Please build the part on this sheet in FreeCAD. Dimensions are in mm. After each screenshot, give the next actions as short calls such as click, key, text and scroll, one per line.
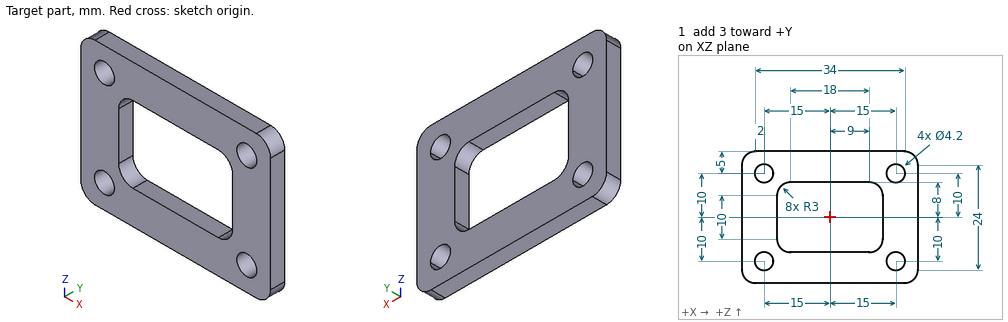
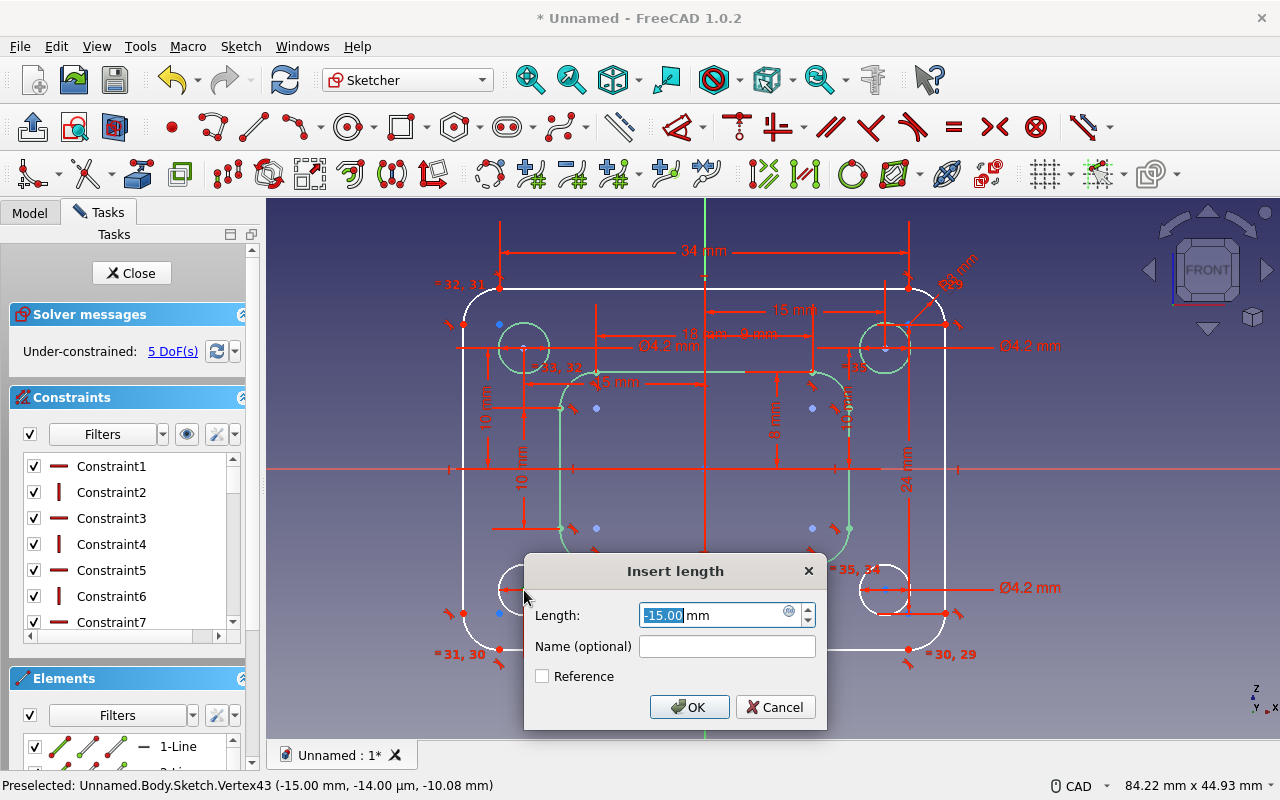
text(-15)
key(Return)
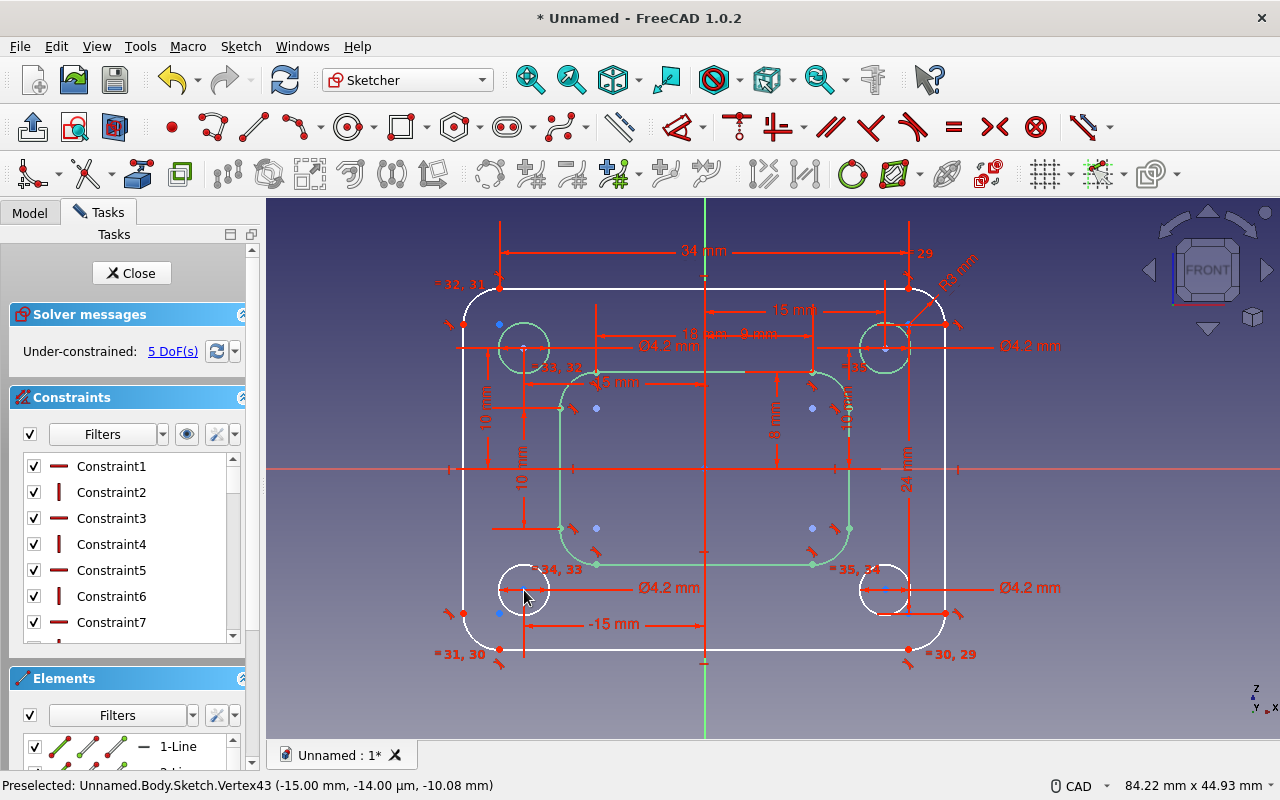
click(524, 590)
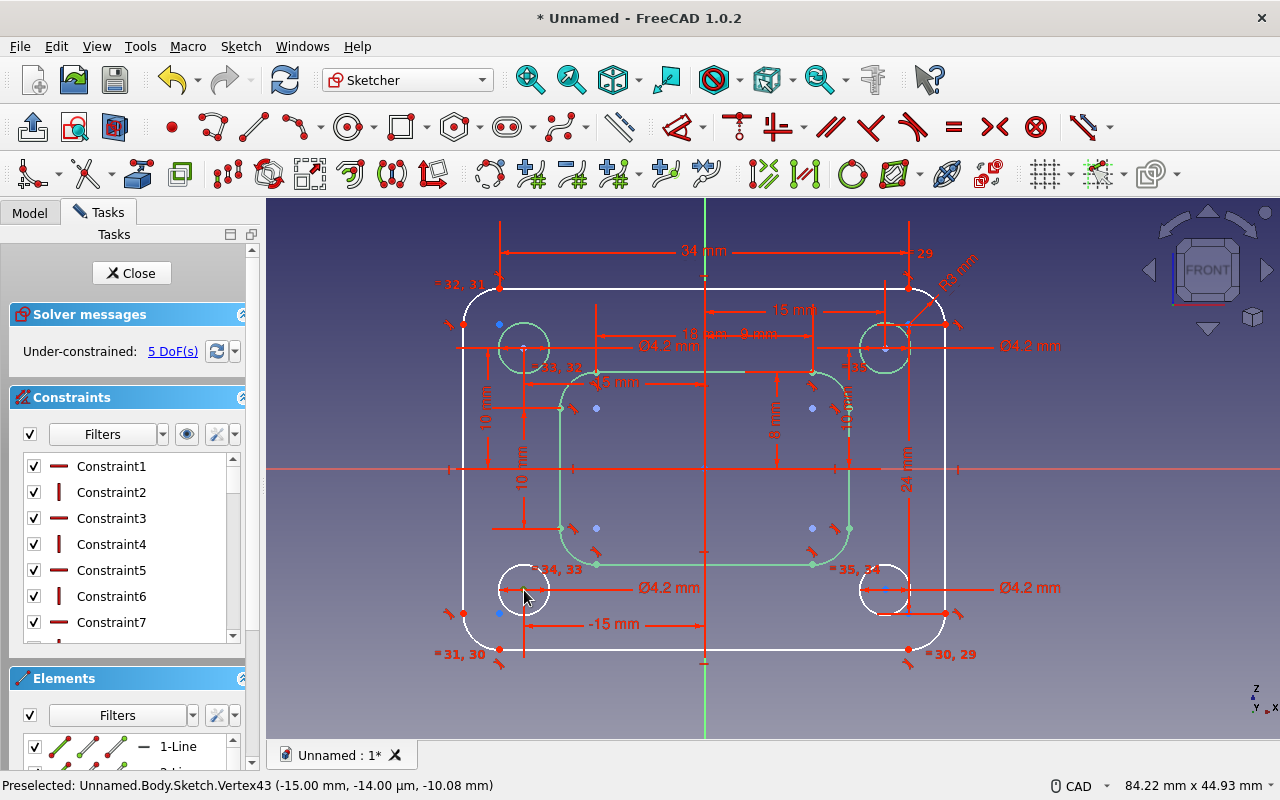
key(i)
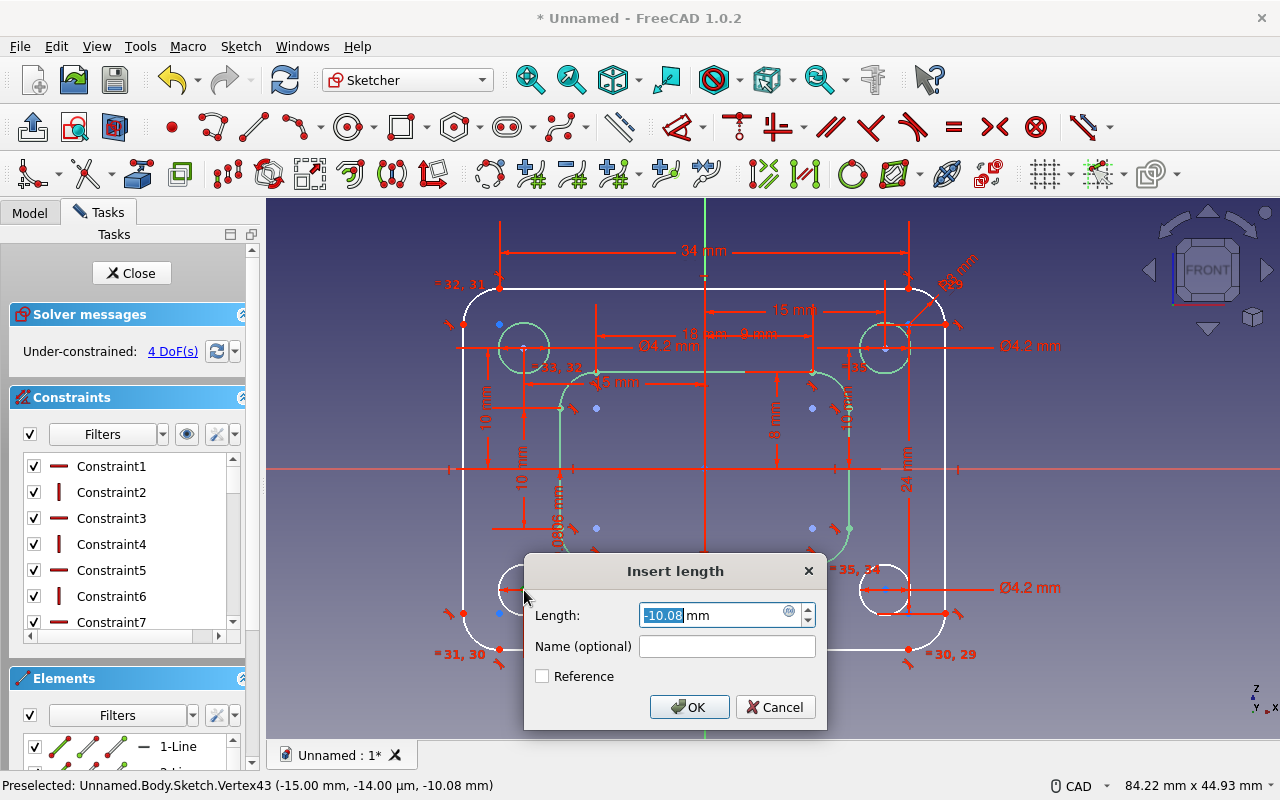
text(-10)
key(Return)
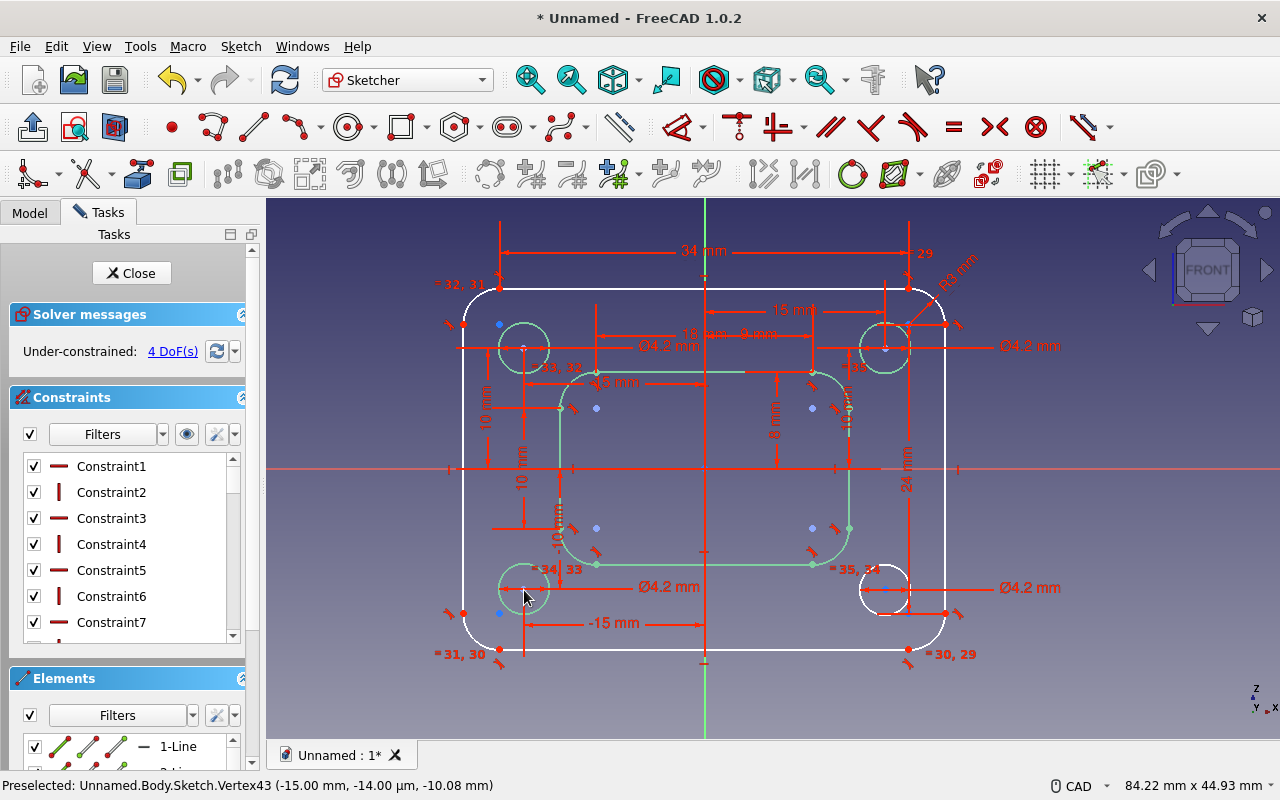
click(885, 590)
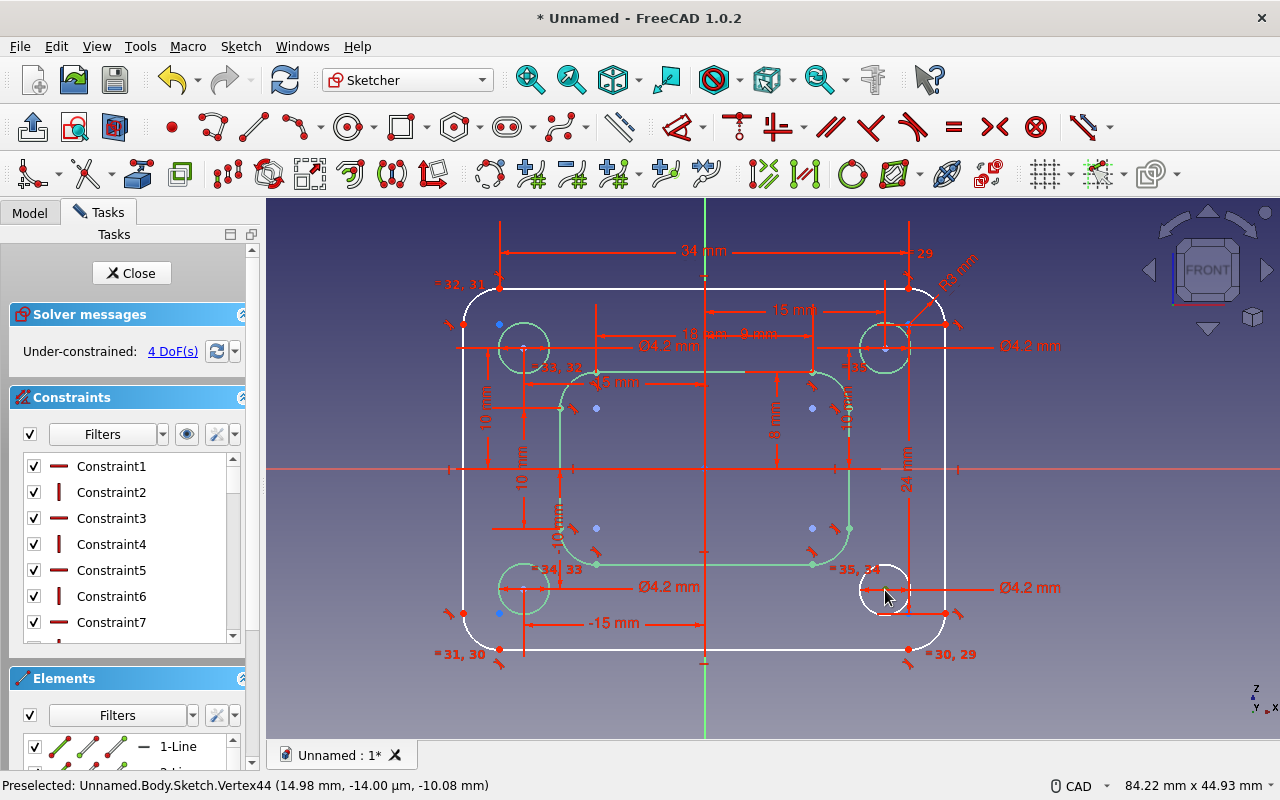
key(l)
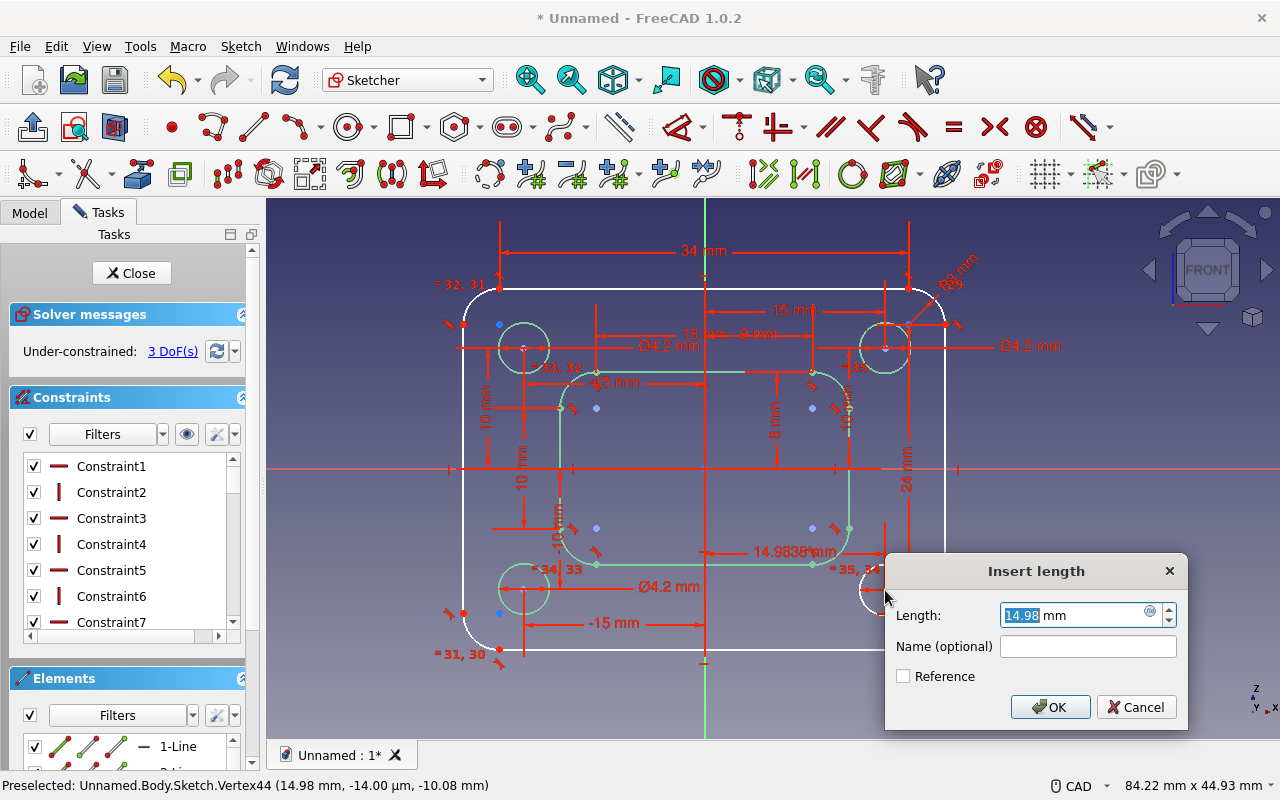
text(15)
key(Return)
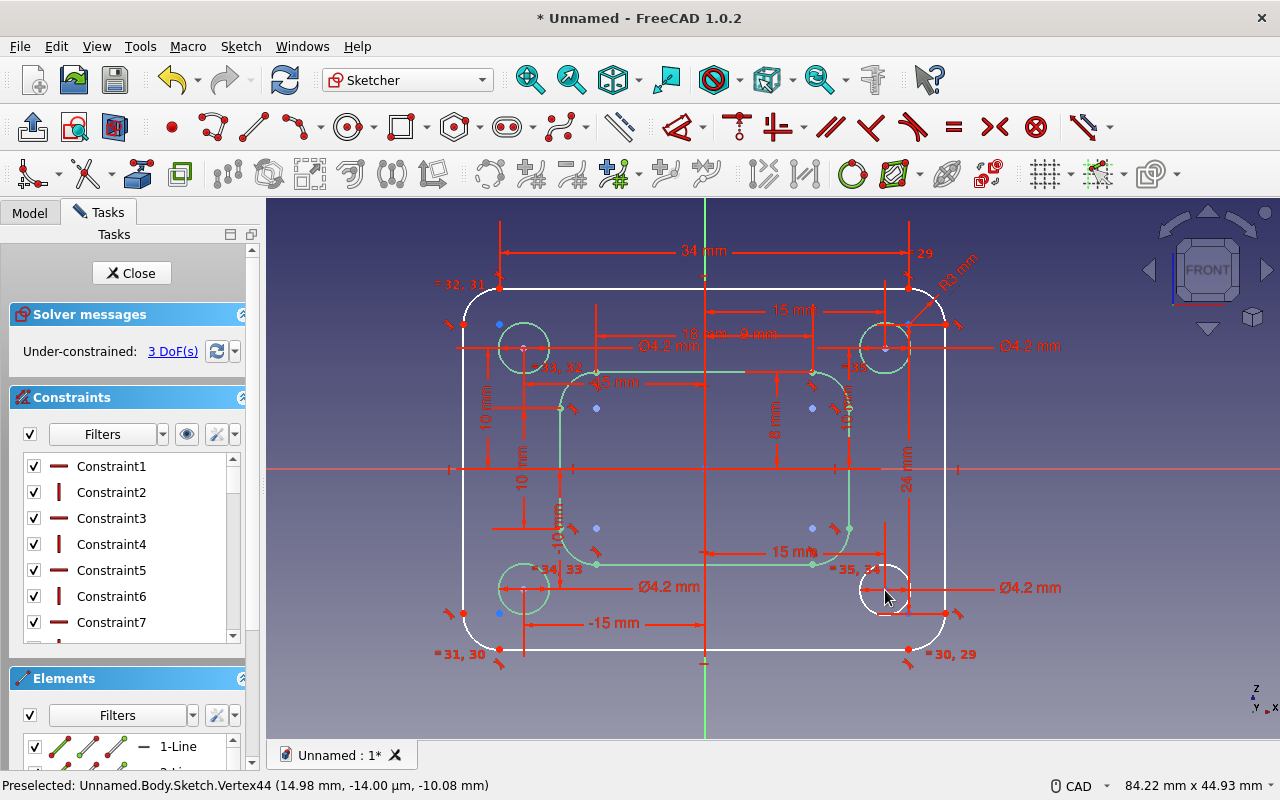
click(885, 590)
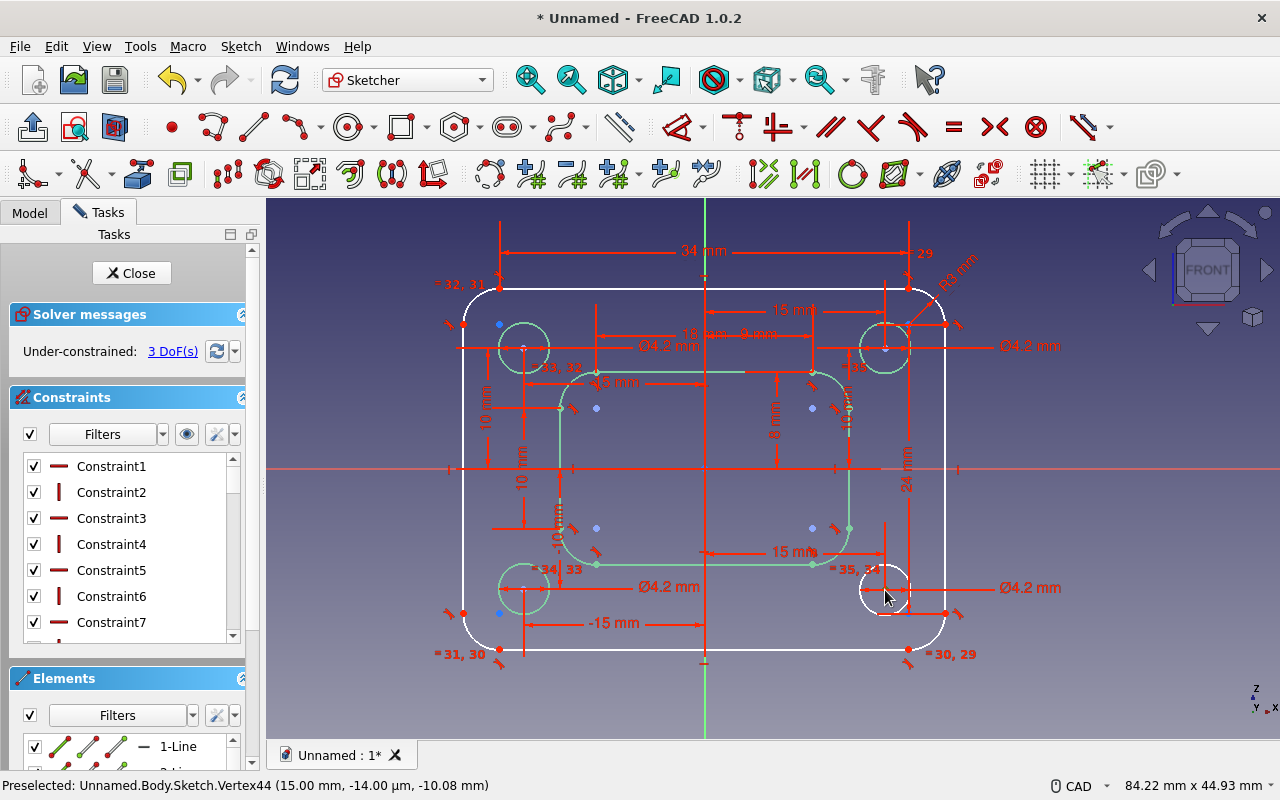
key(i)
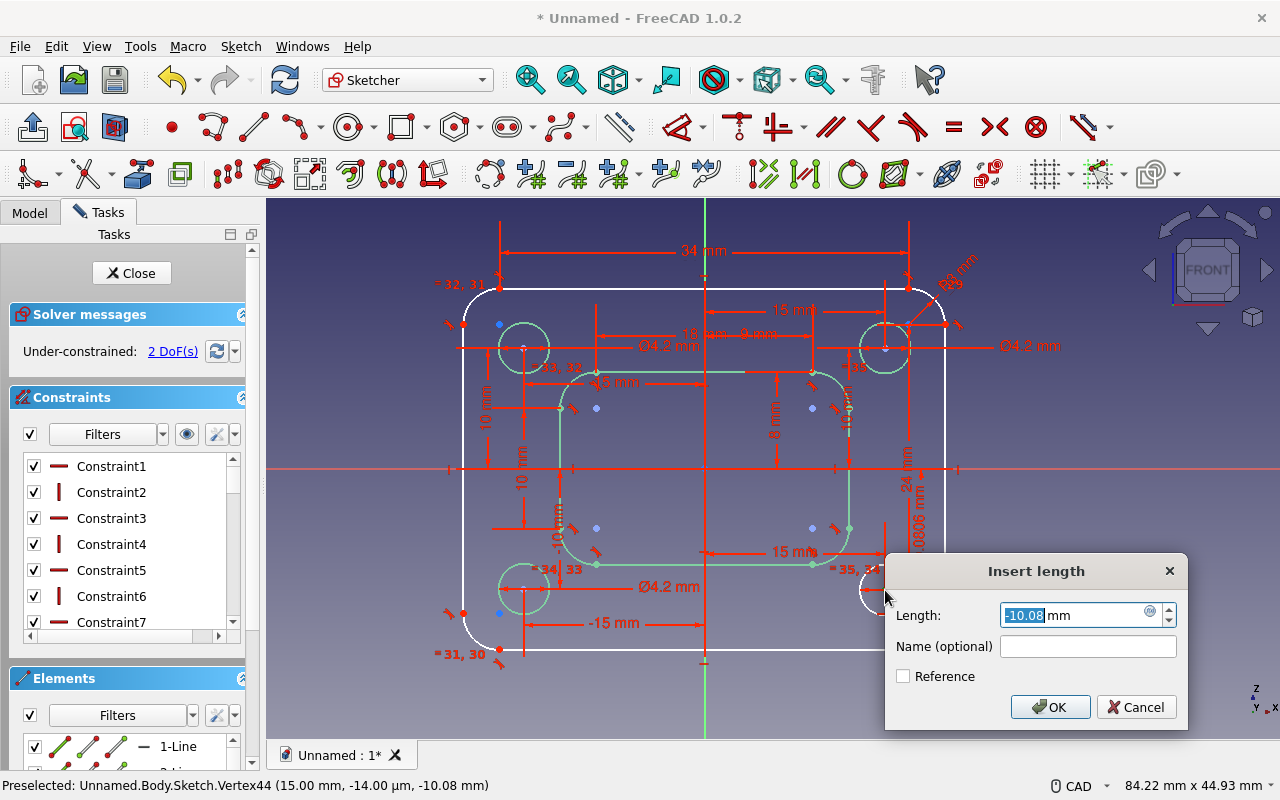
text(-10)
key(Return)